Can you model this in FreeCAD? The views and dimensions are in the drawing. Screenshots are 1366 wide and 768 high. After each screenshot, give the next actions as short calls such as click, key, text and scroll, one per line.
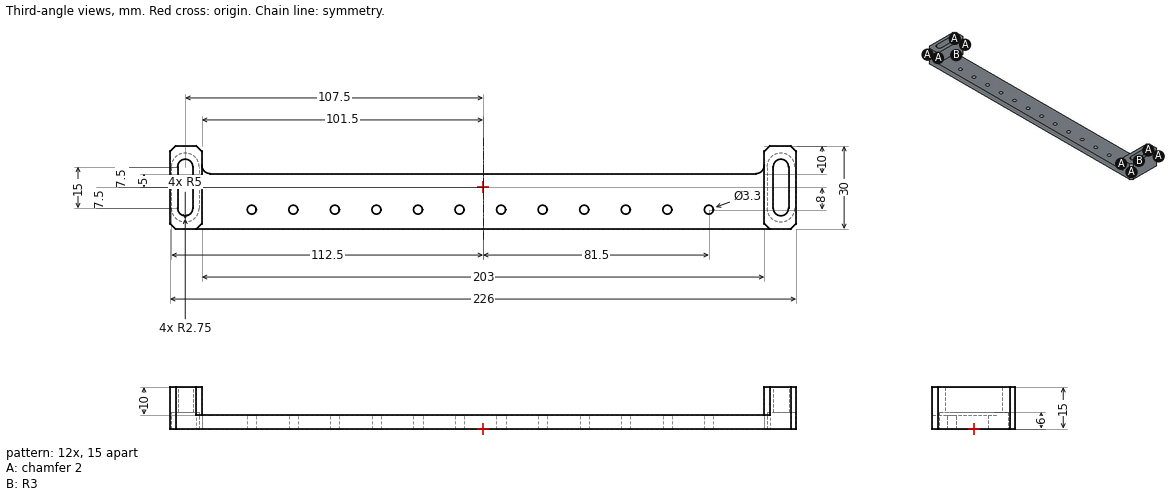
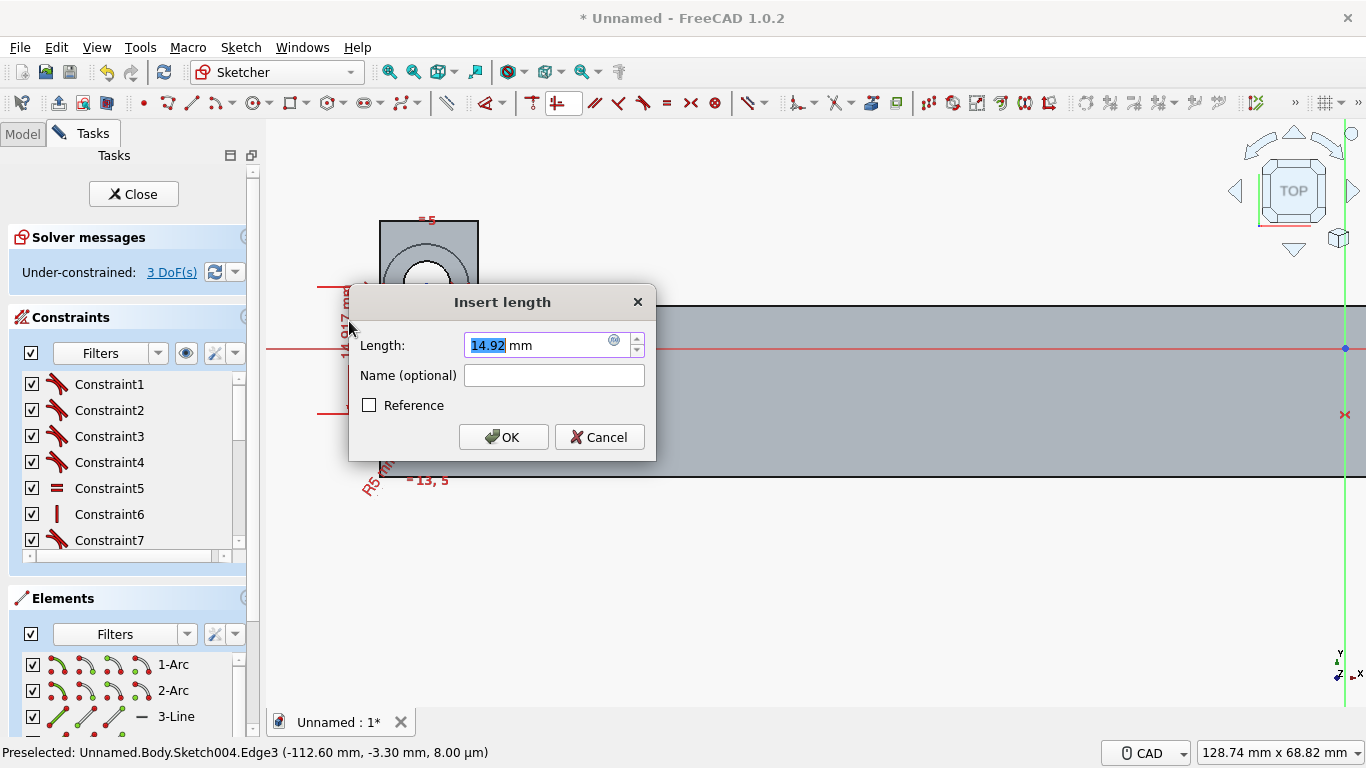
text(15)
key(Return)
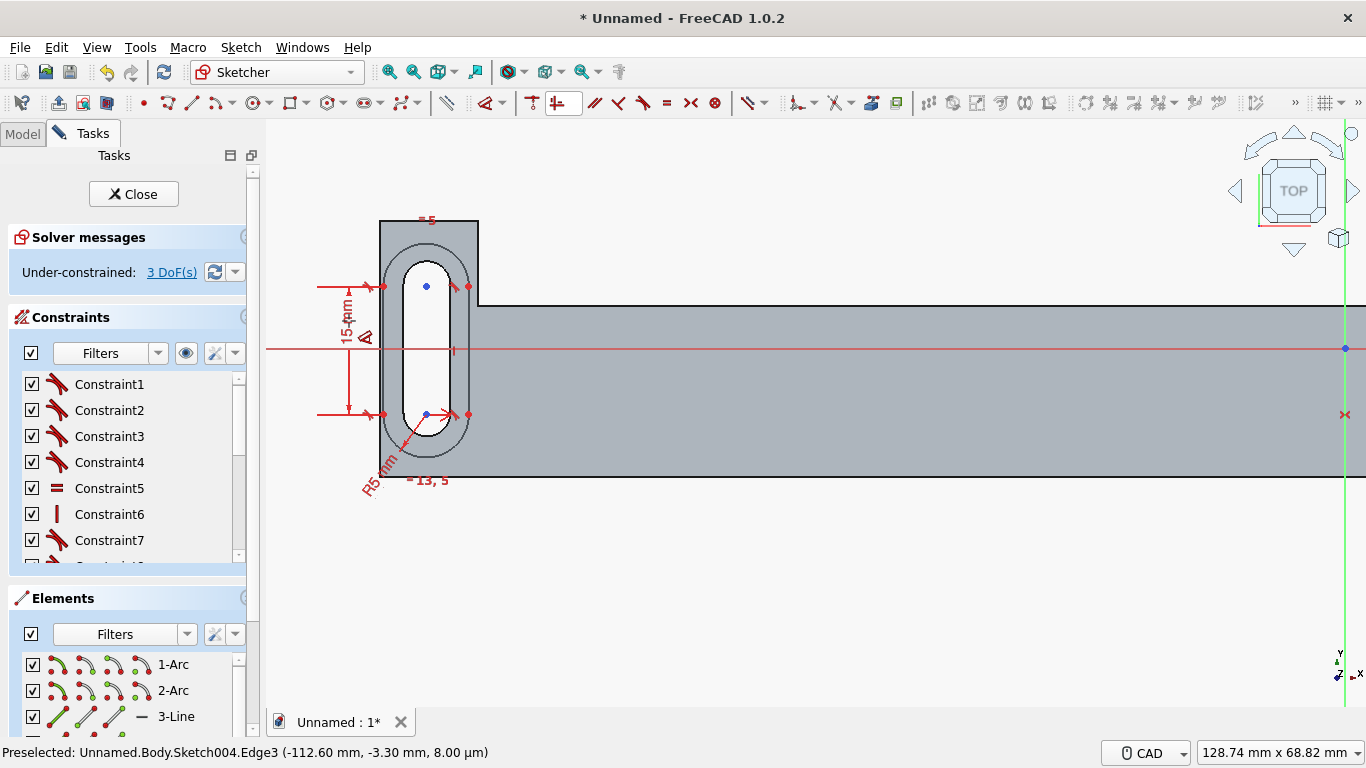
scroll(399, 450, down, 5)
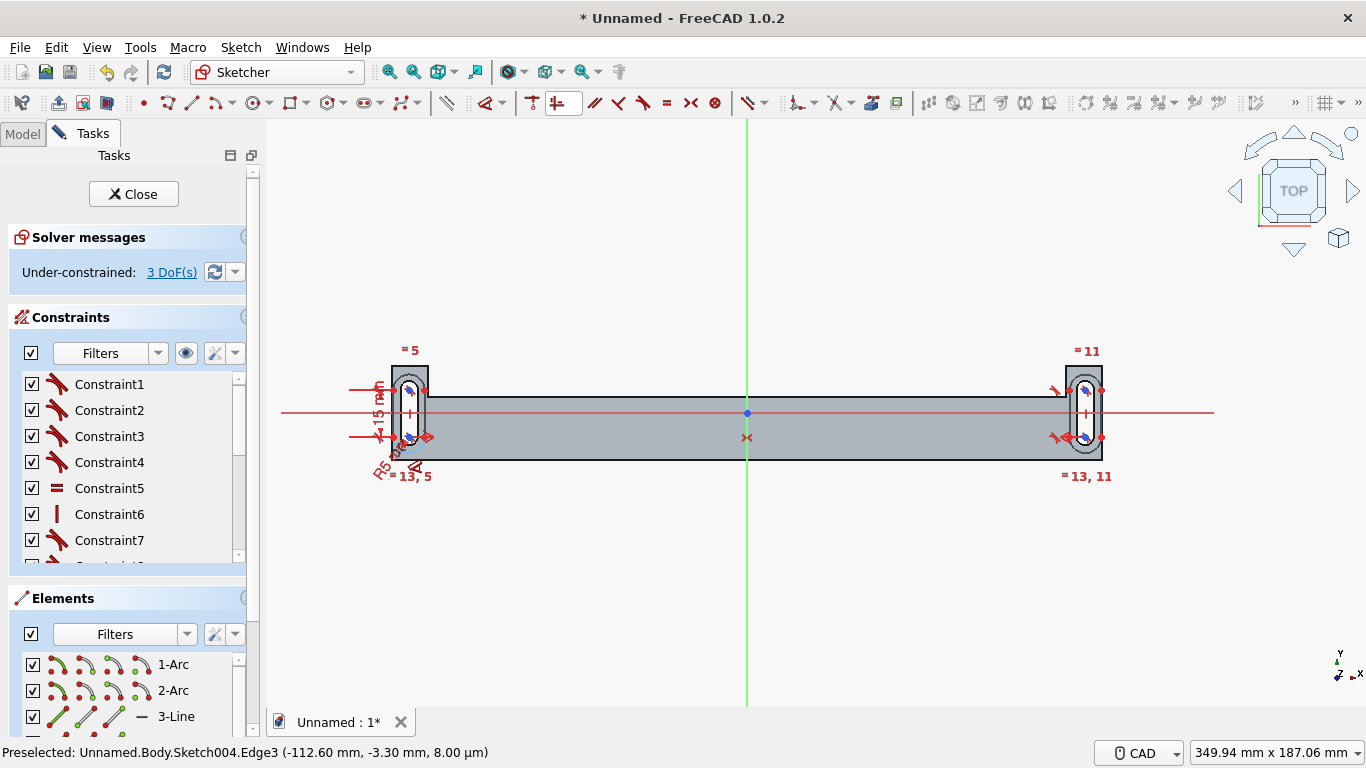
scroll(1070, 423, up, 2)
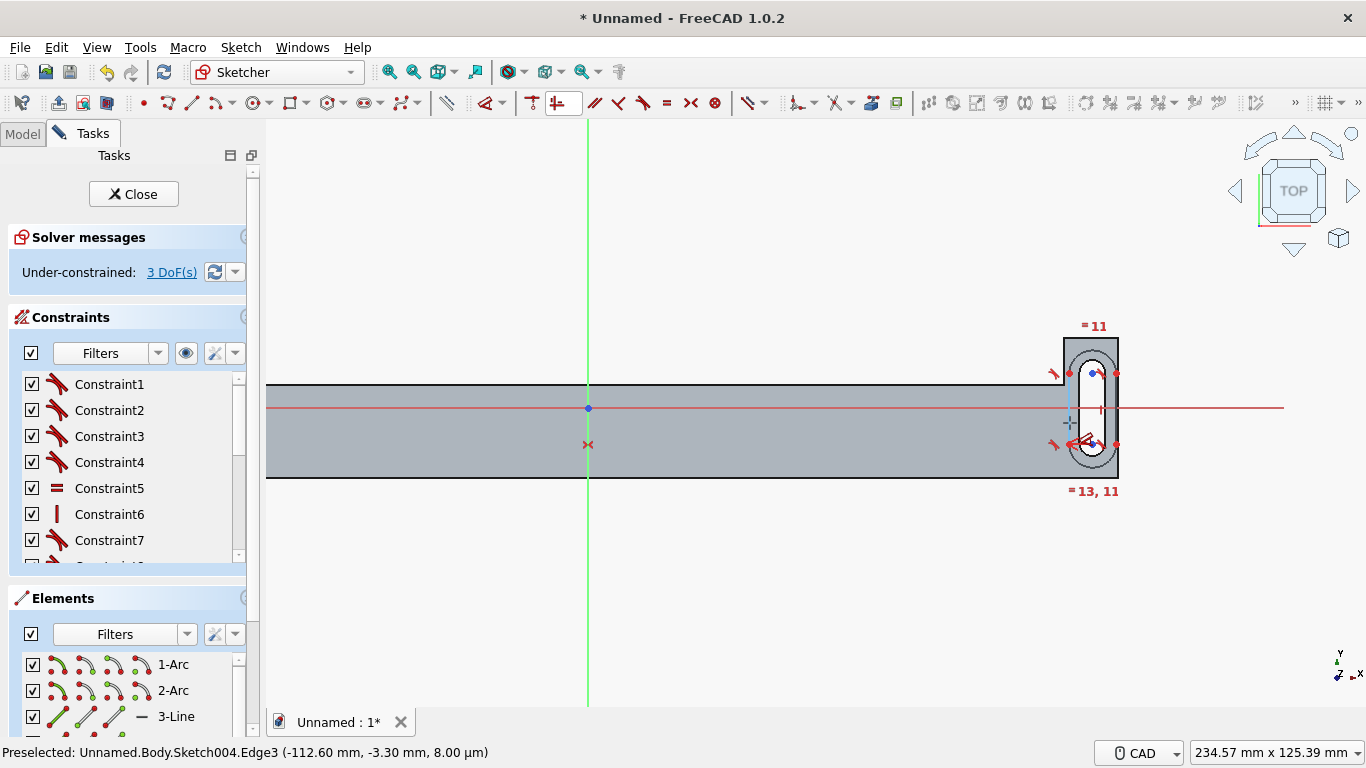
click(1069, 423)
click(1035, 393)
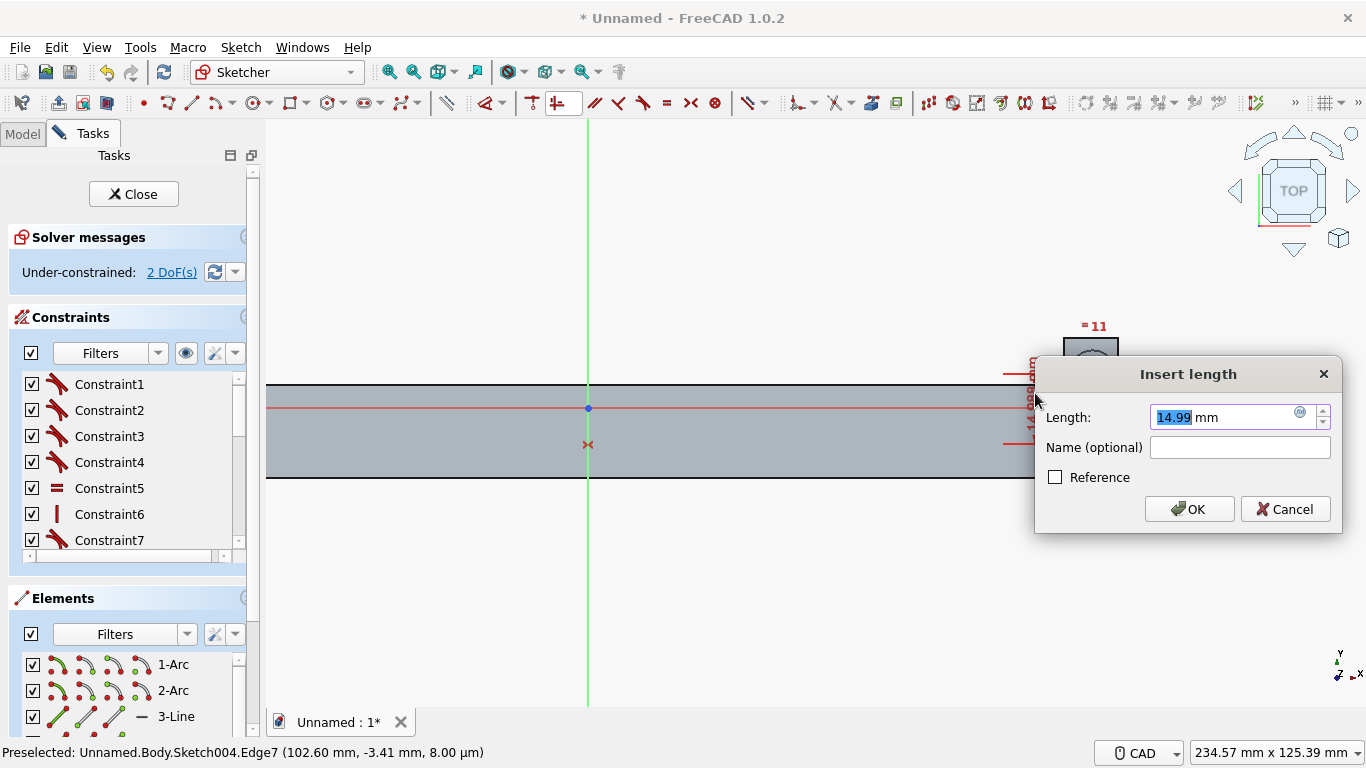
text(15)
key(Return)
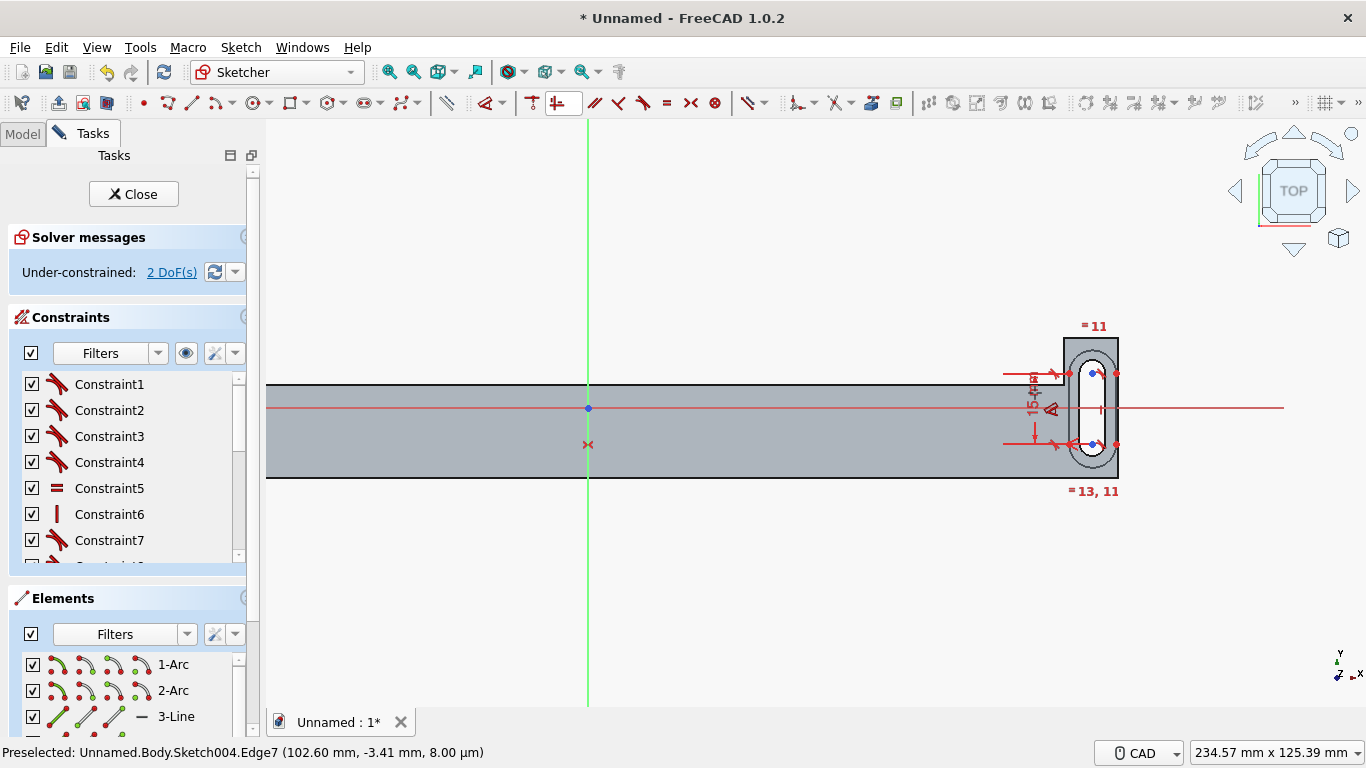
scroll(1071, 423, down, 2)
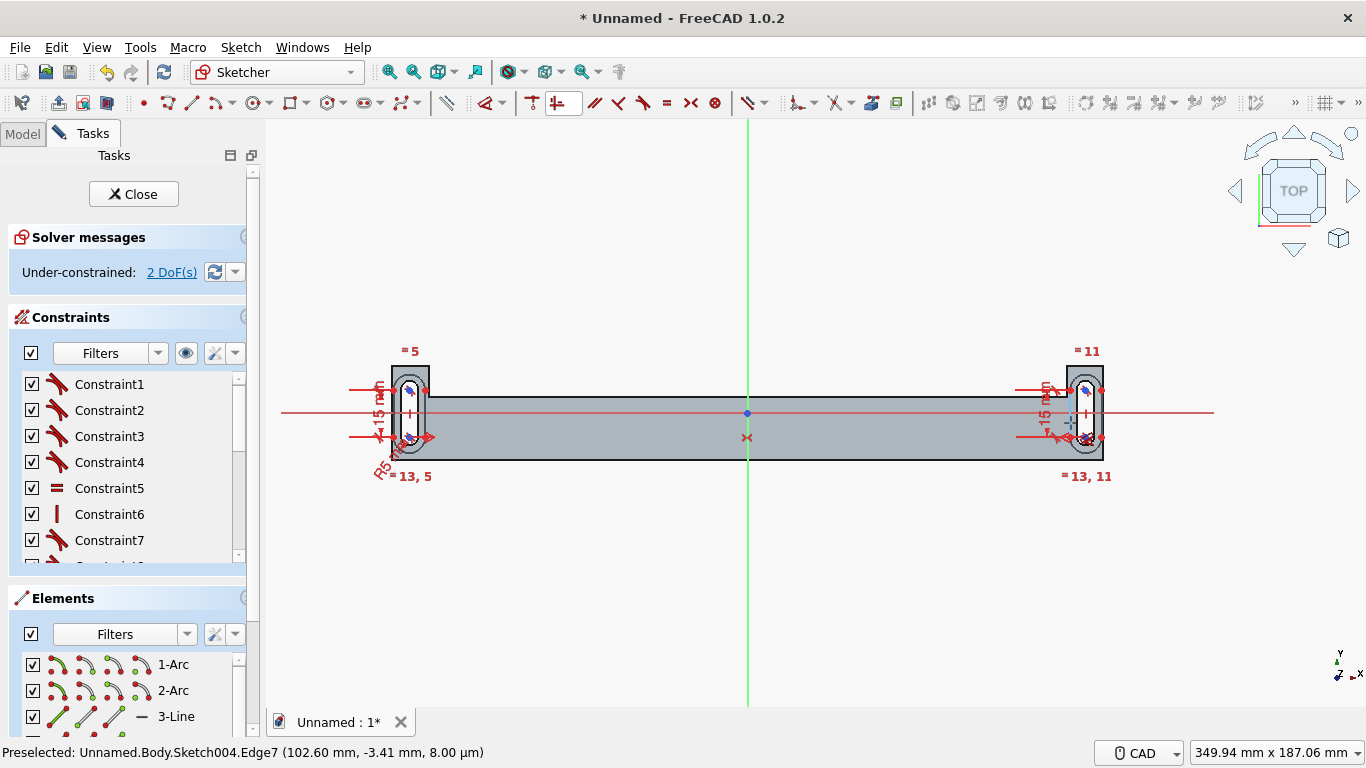
scroll(394, 437, up, 3)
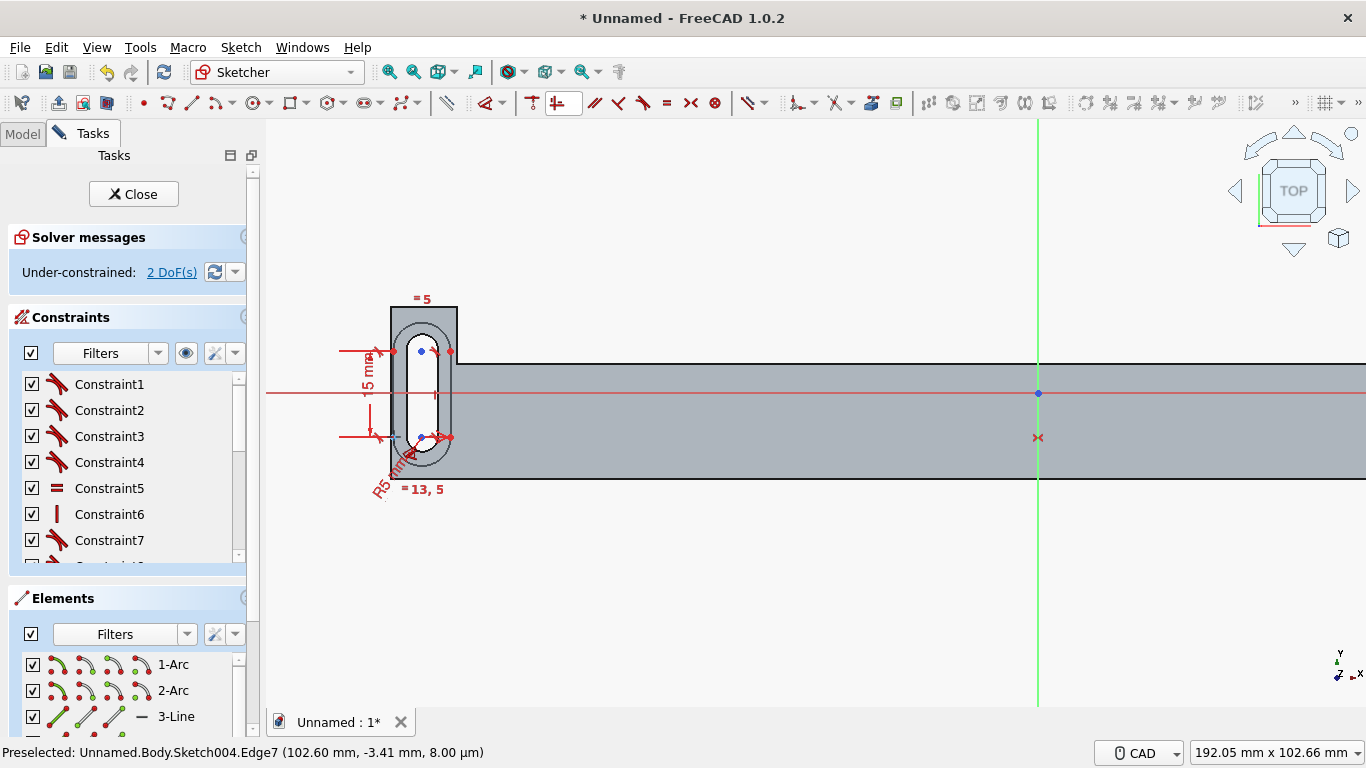
click(393, 437)
click(359, 415)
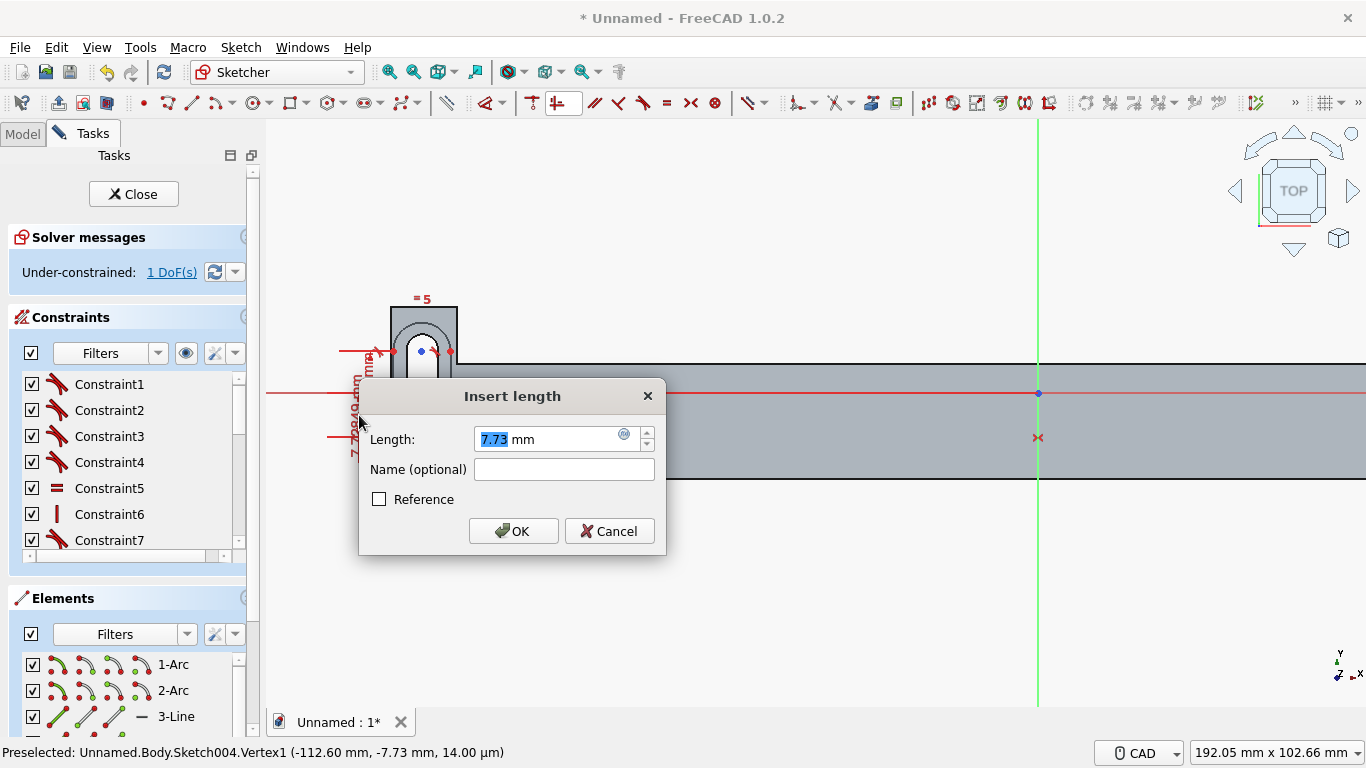
text(7.5)
key(Return)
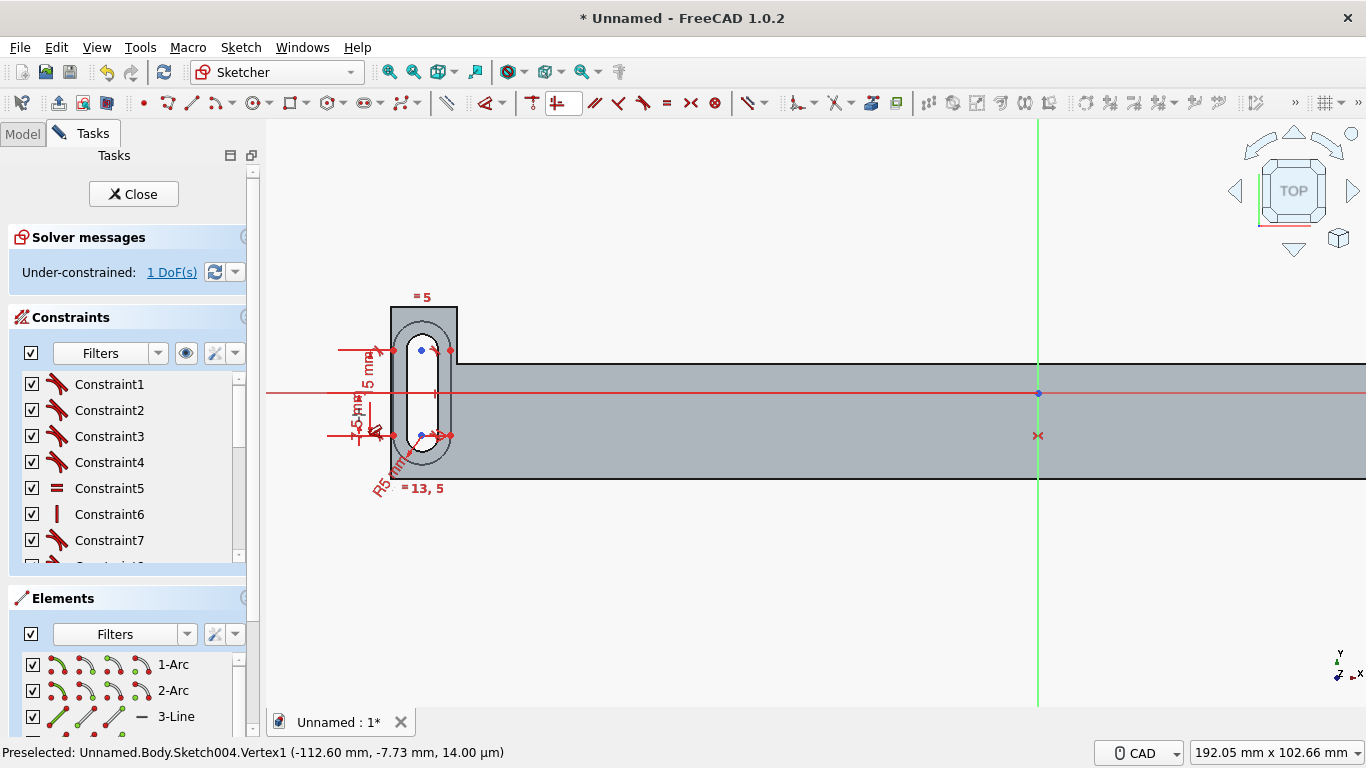
click(393, 436)
click(716, 470)